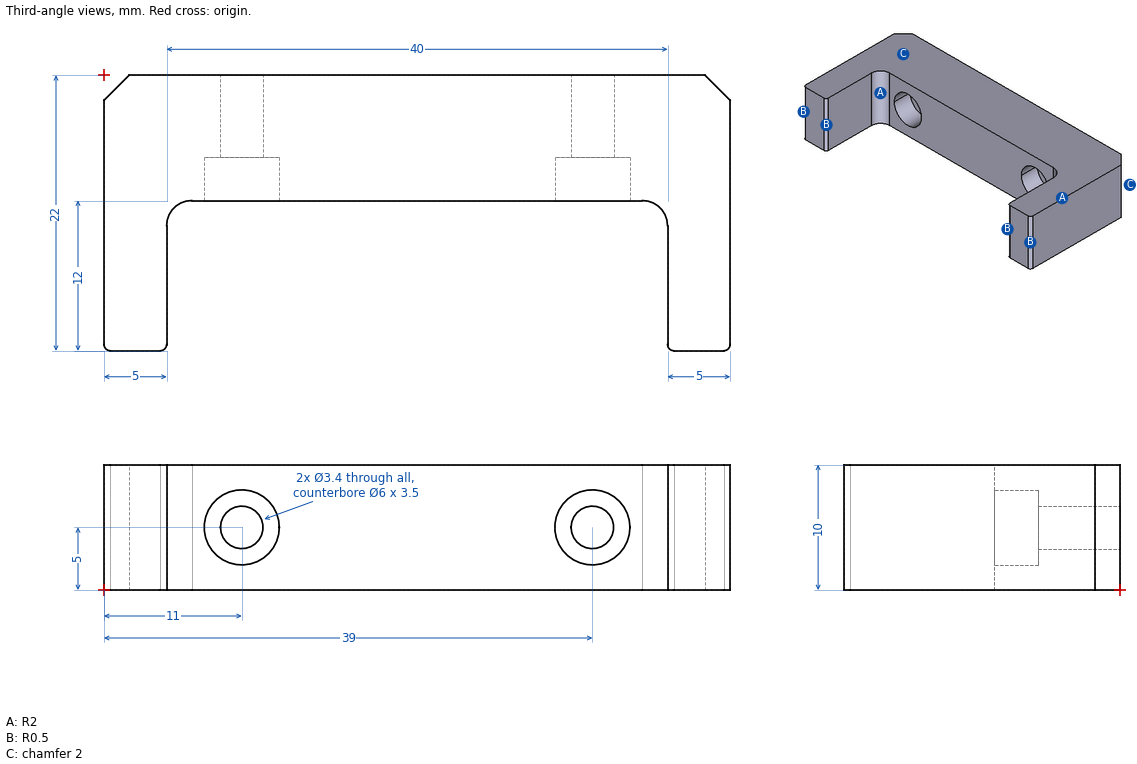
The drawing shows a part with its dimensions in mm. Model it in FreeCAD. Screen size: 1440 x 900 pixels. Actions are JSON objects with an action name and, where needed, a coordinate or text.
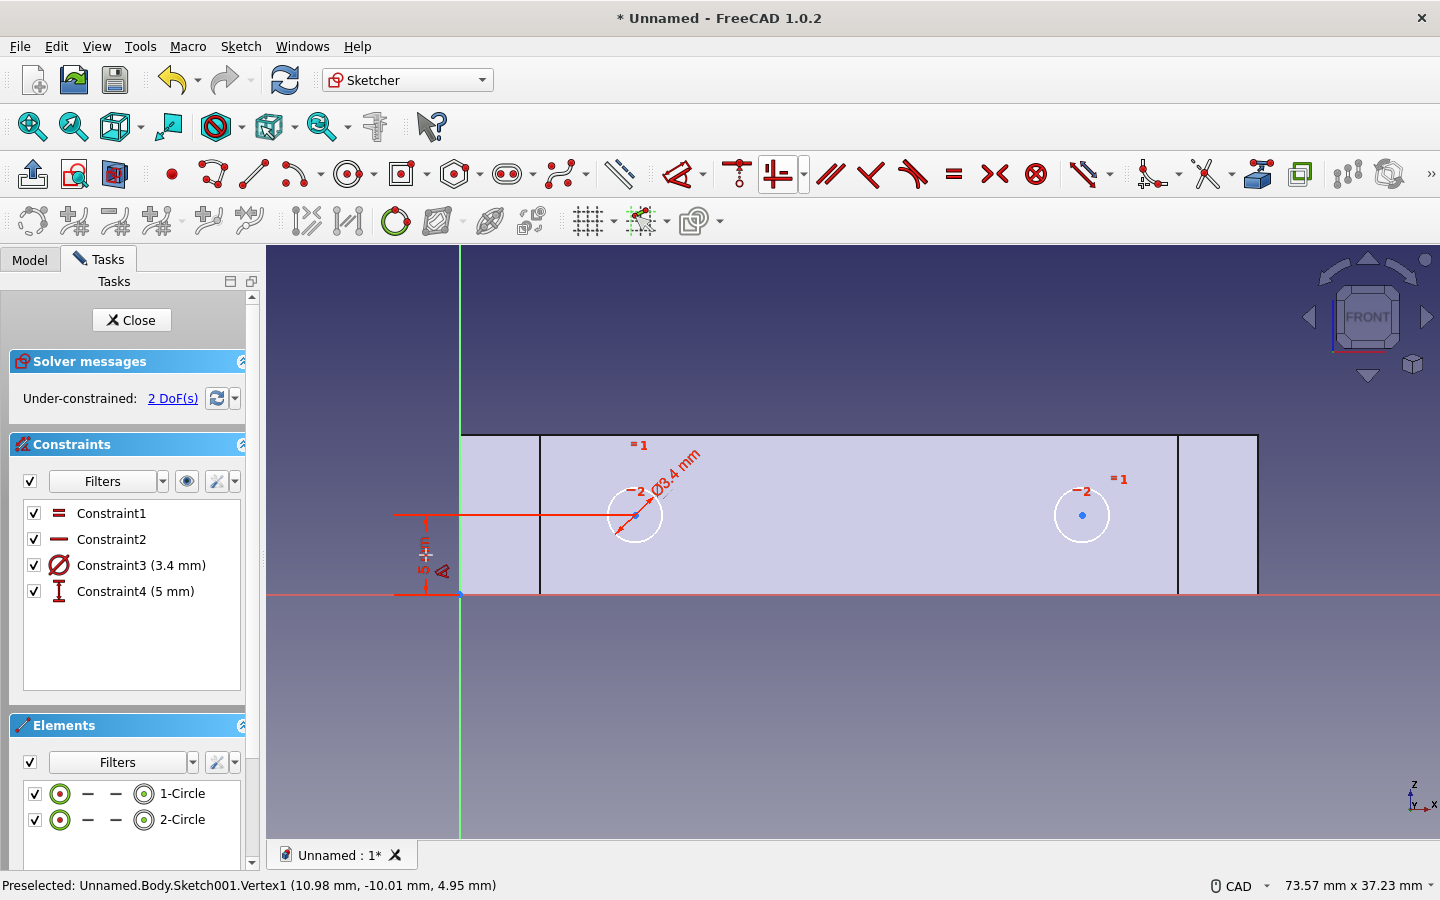
{"action": "left_click", "coordinate": [635, 515]}
{"action": "left_click", "coordinate": [547, 629]}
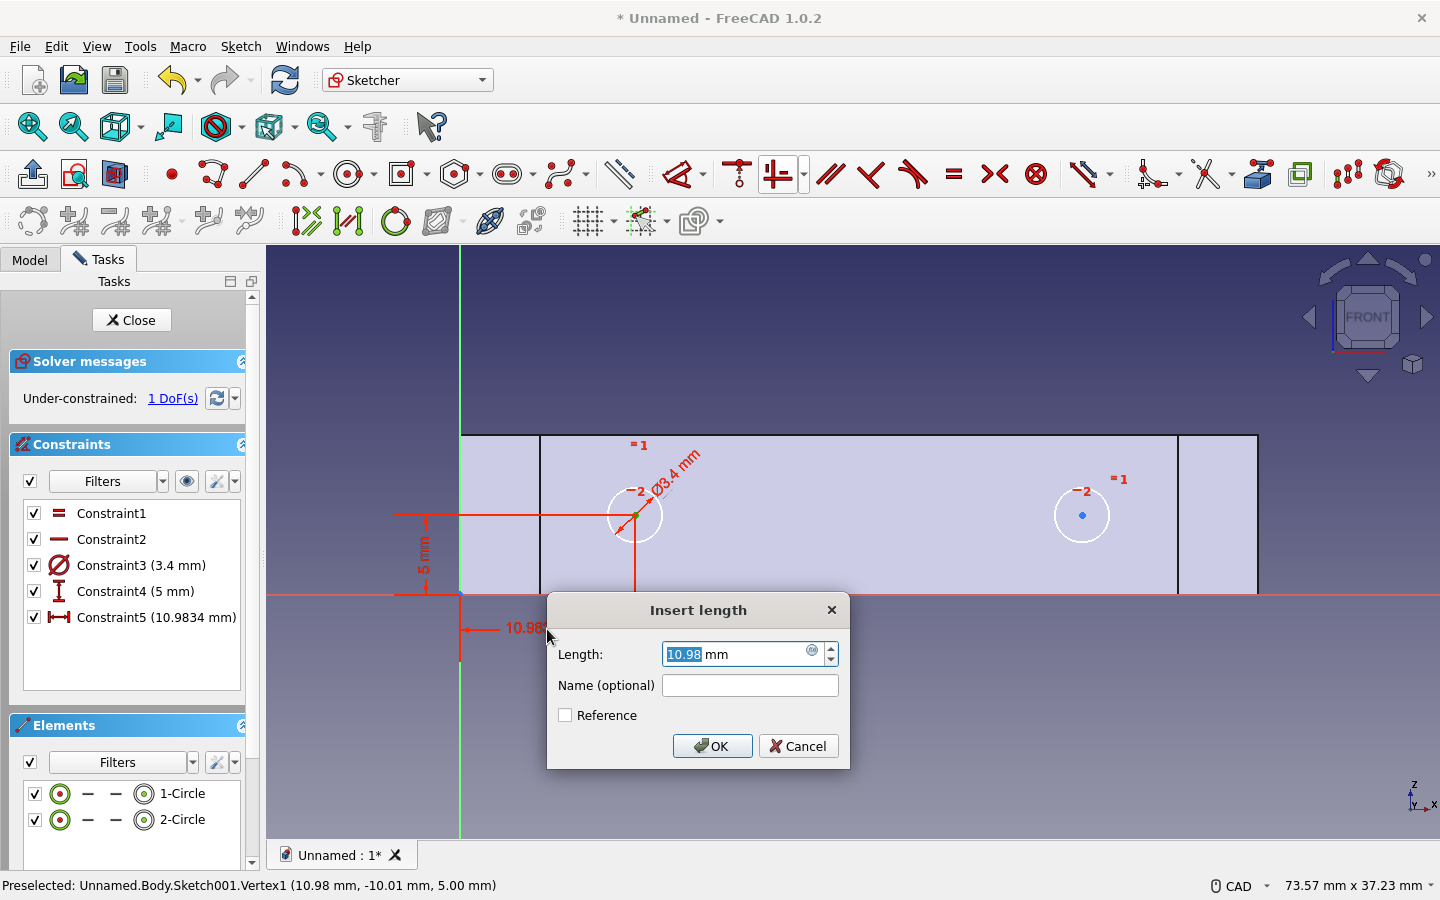
{"action": "type", "text": "11"}
{"action": "key", "text": "Return"}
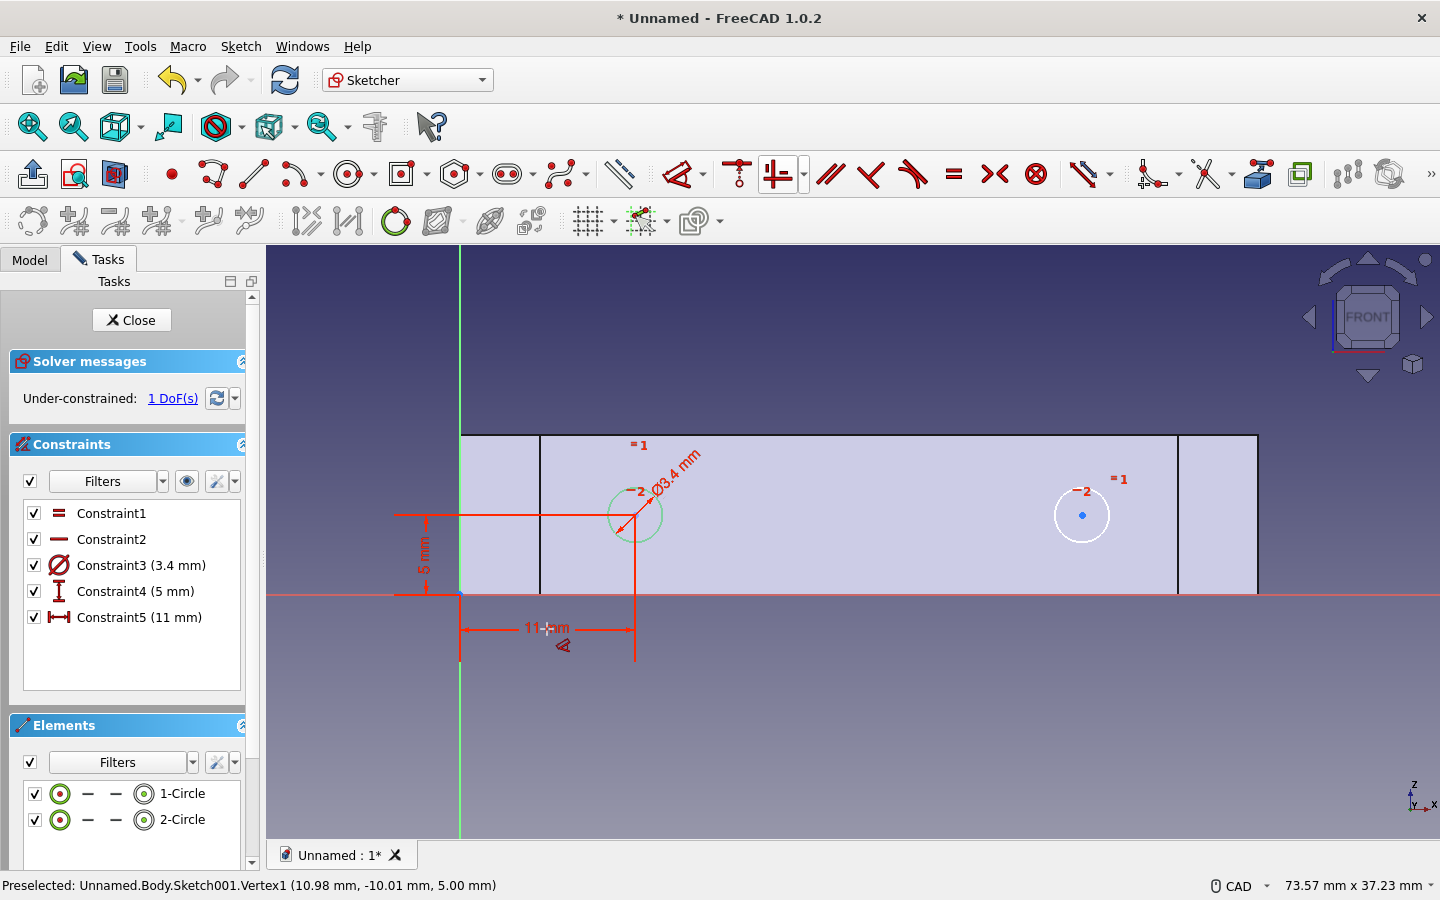
{"action": "left_click", "coordinate": [1082, 515]}
{"action": "left_click", "coordinate": [771, 629]}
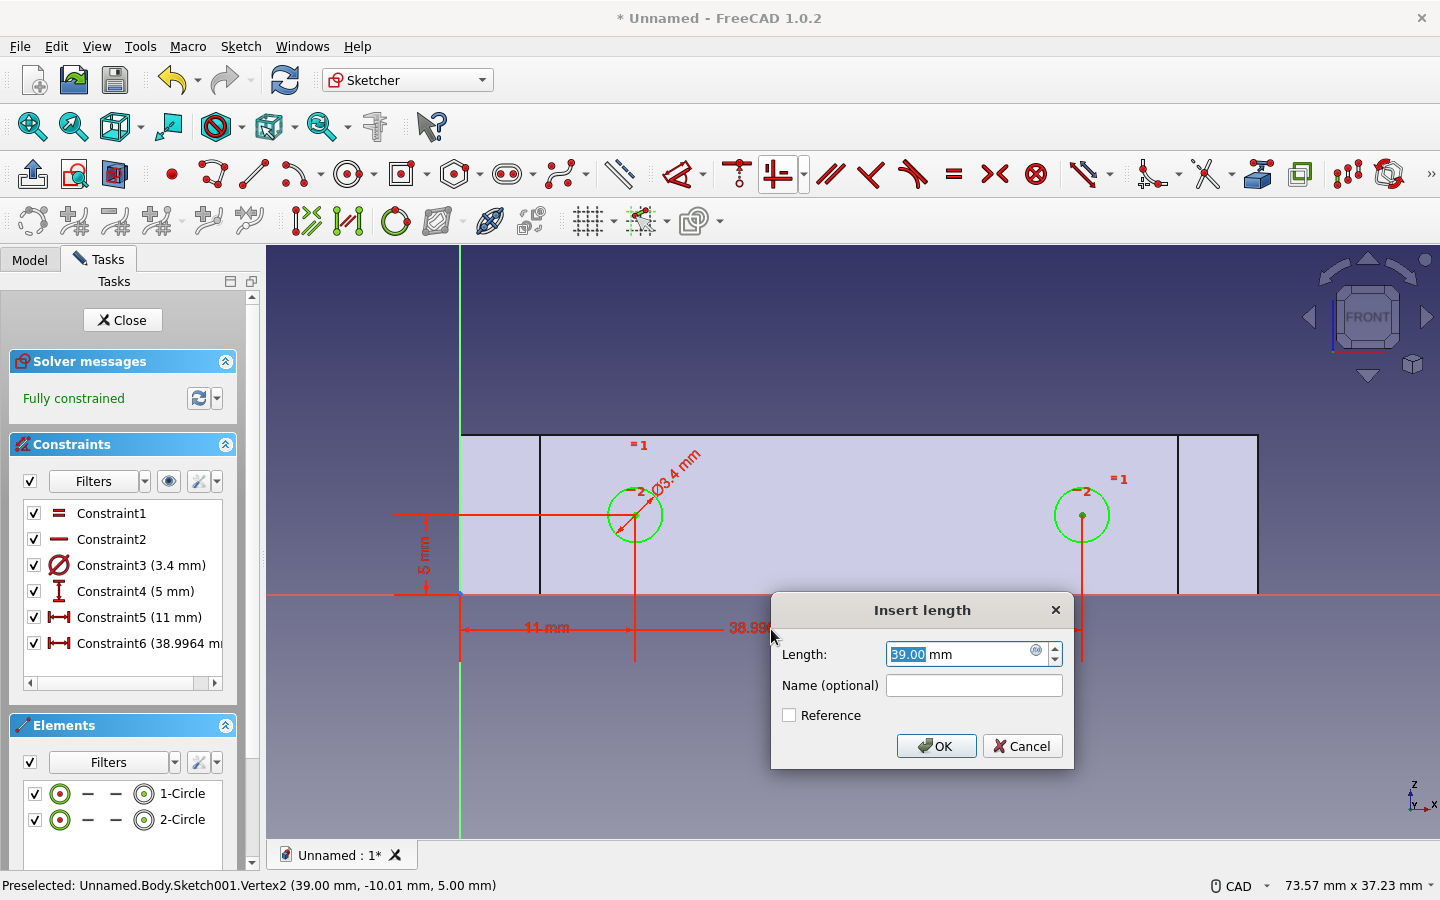
{"action": "type", "text": "39"}
{"action": "key", "text": "Return"}
{"action": "key", "text": "Escape"}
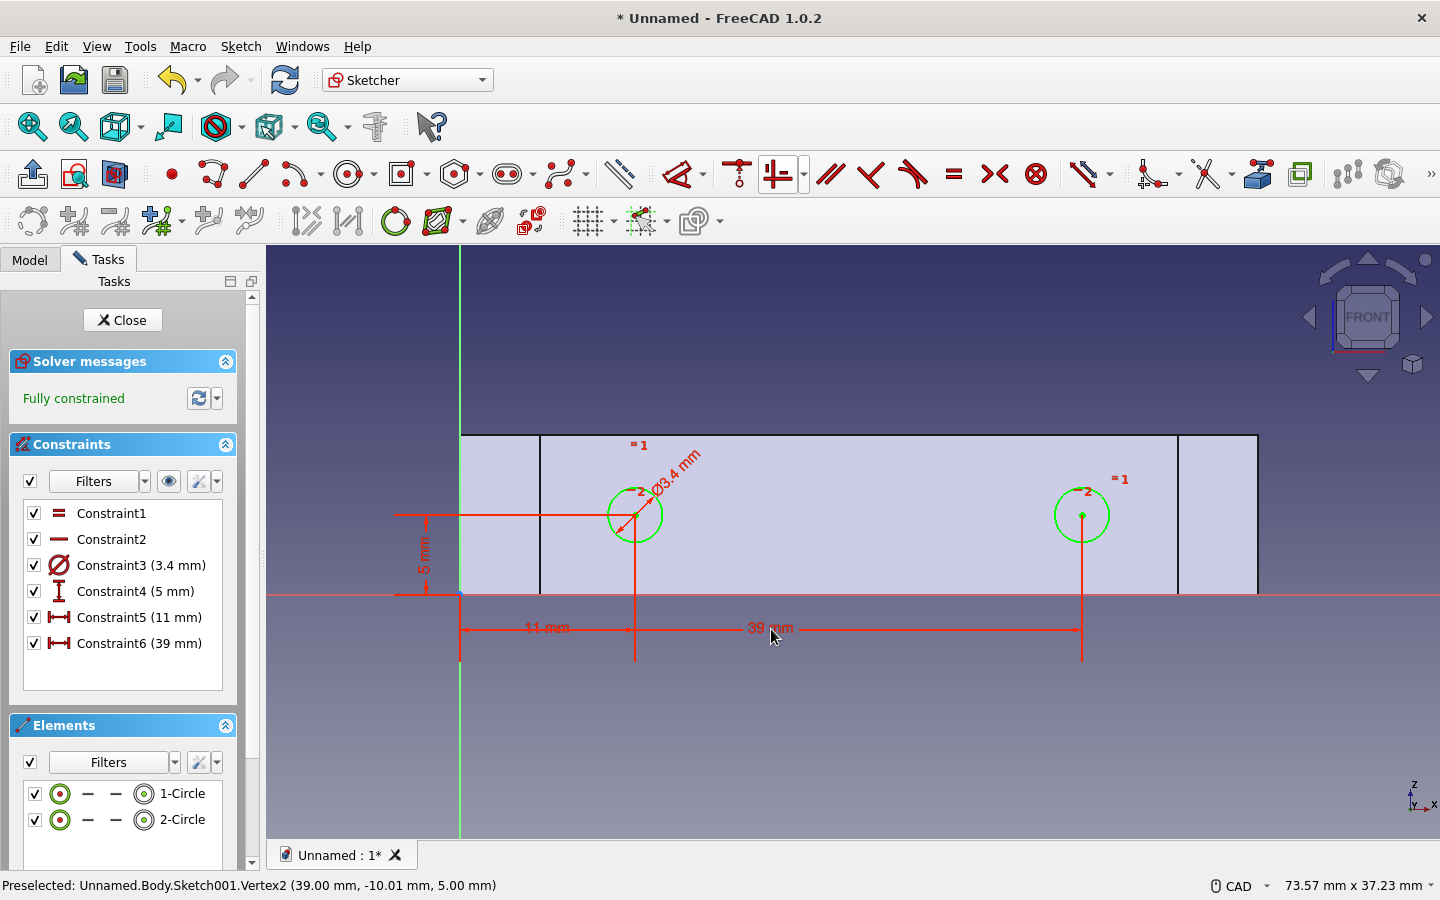
{"action": "left_click", "coordinate": [123, 320]}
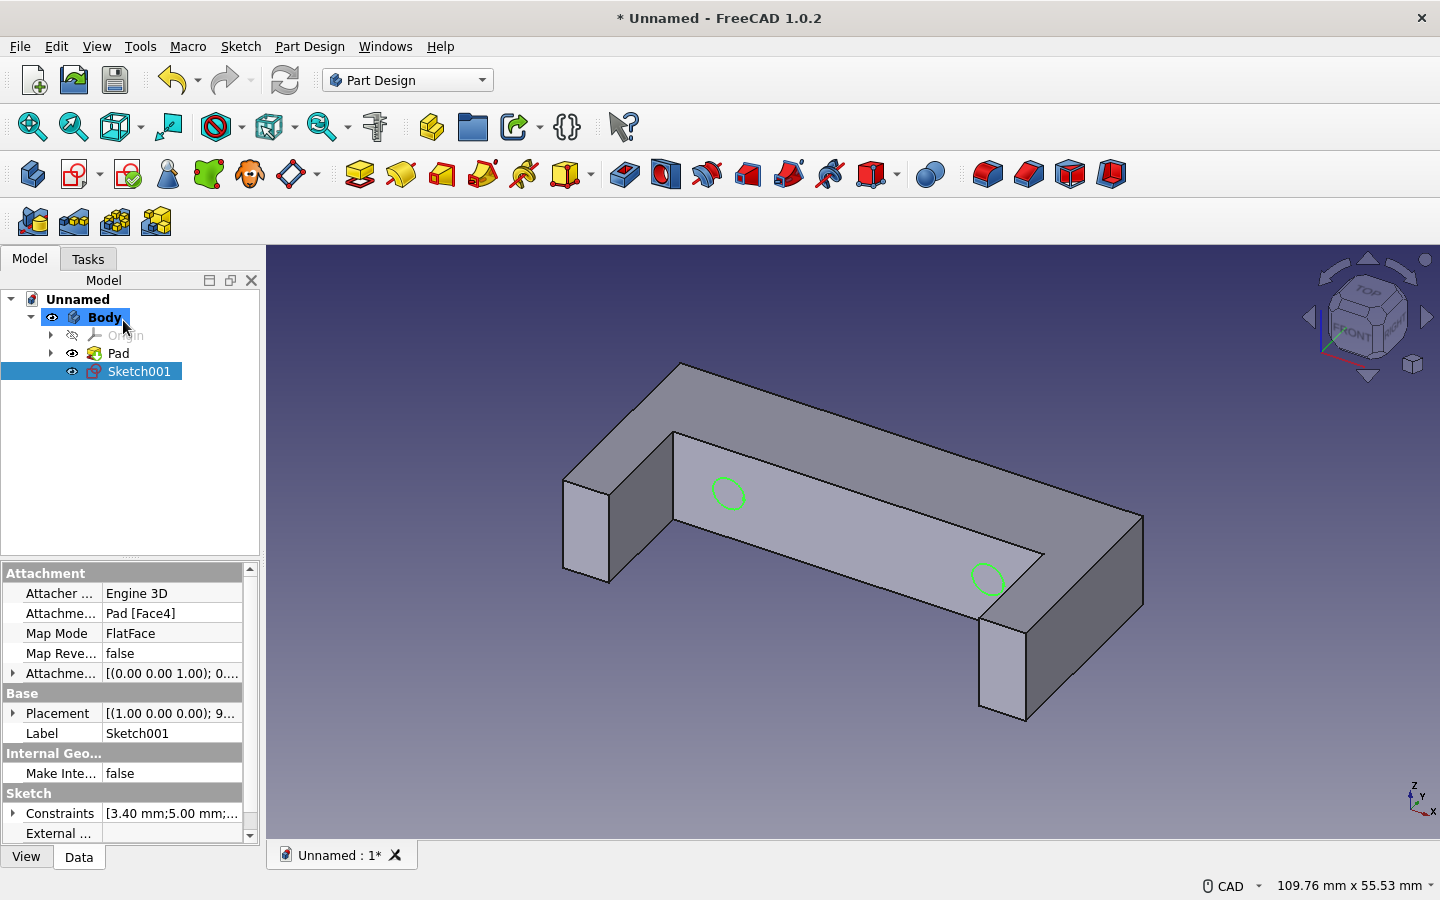
{"action": "left_click", "coordinate": [666, 174]}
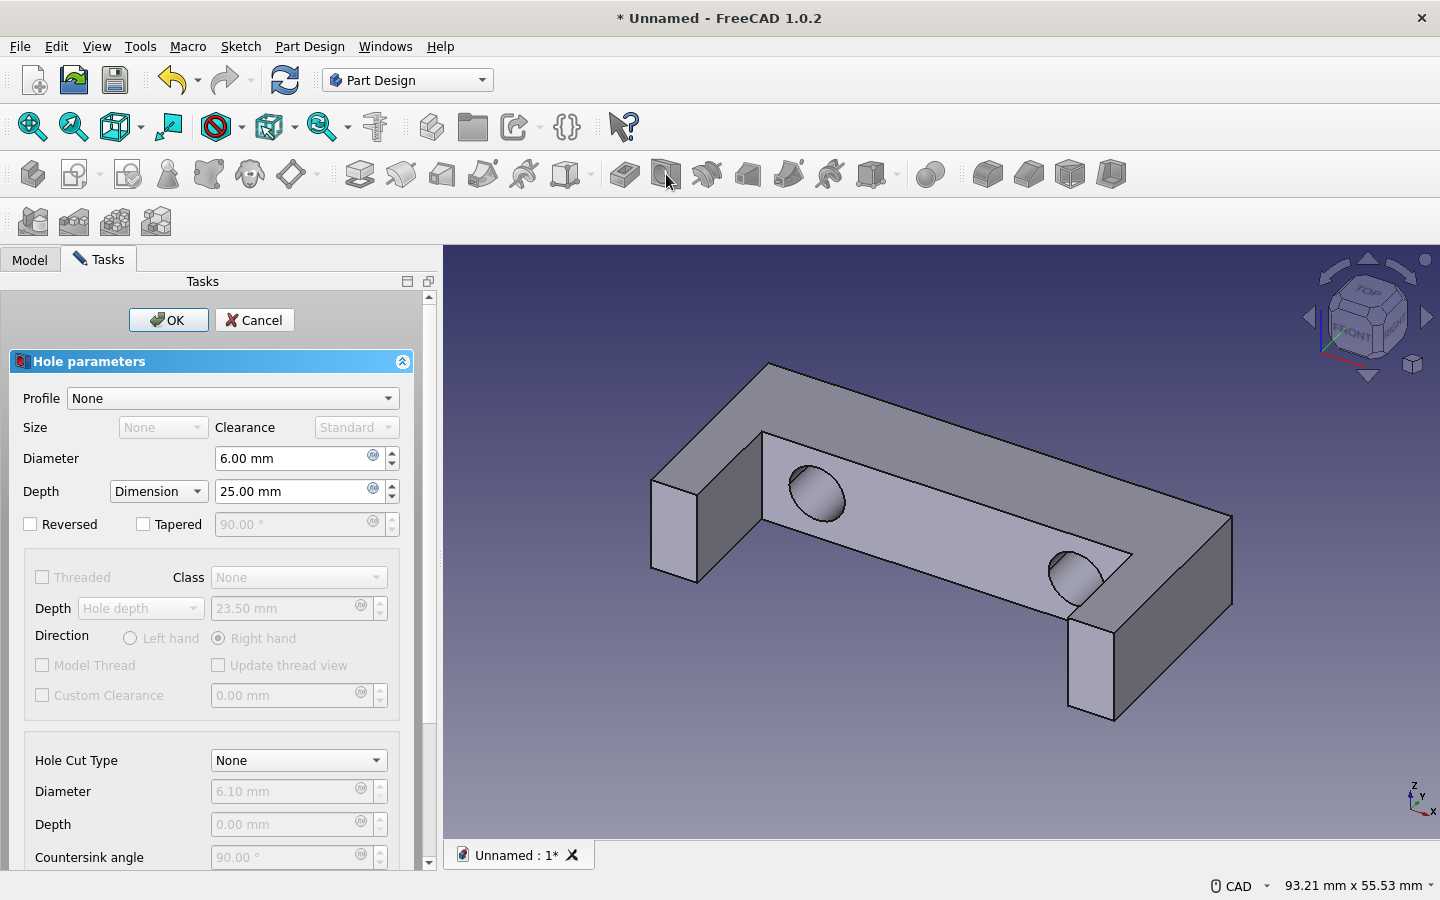
{"action": "triple_click", "coordinate": [300, 458]}